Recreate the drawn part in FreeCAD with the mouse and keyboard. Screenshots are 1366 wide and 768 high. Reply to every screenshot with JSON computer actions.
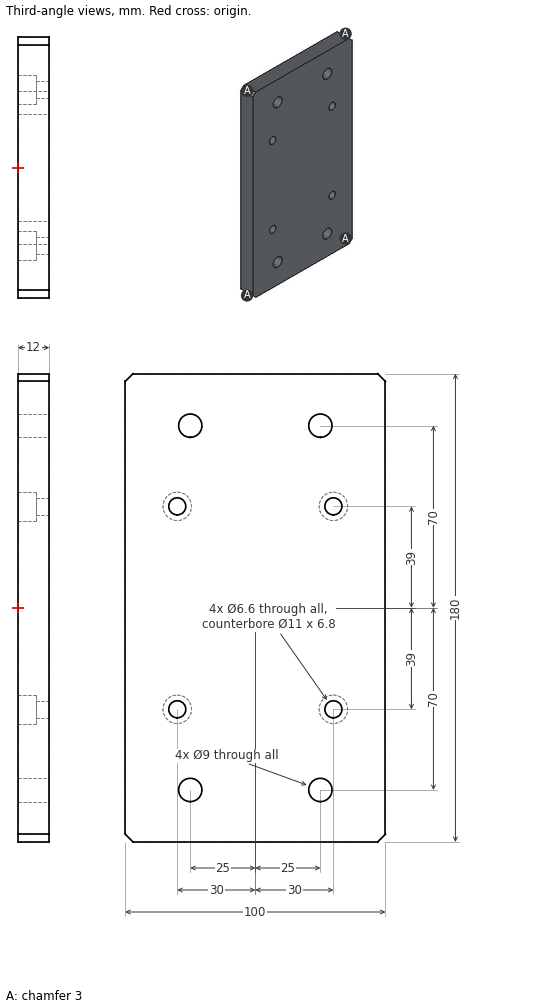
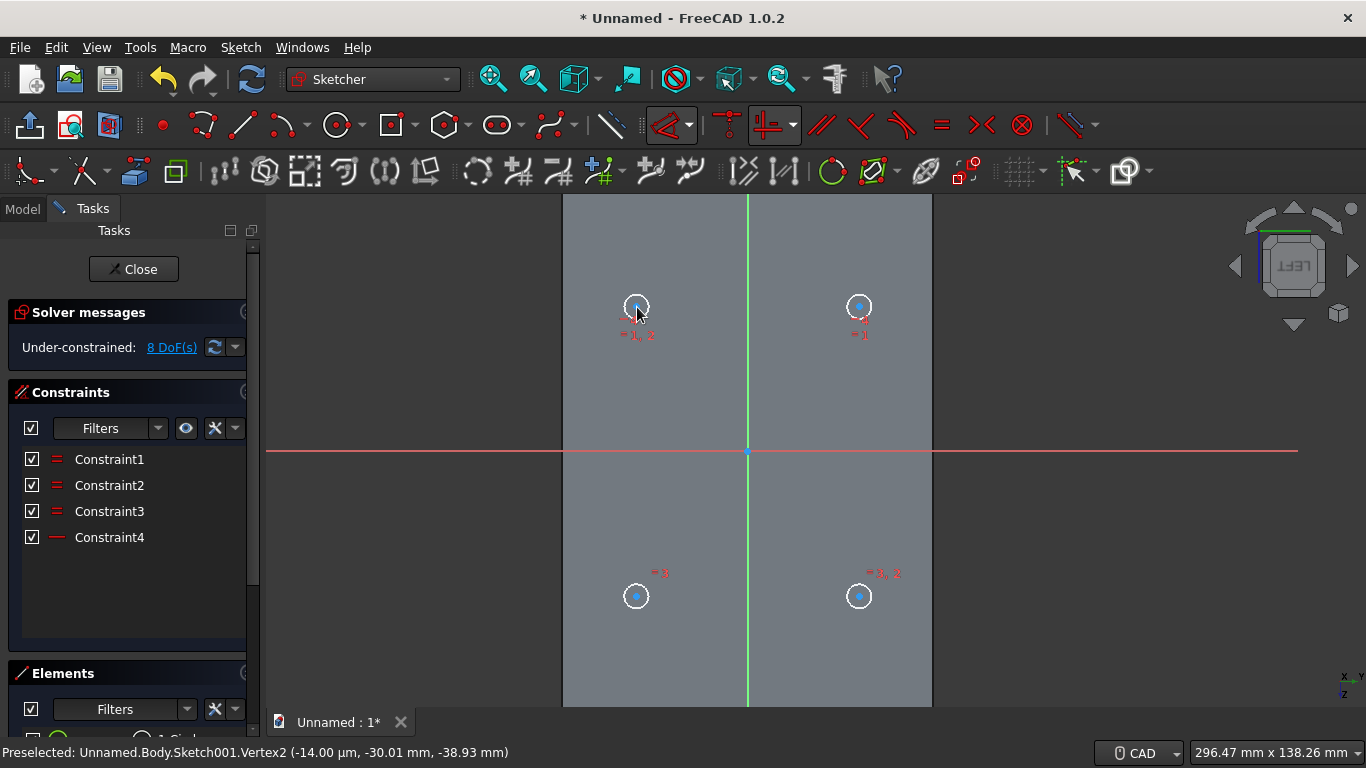
{"action": "left_click", "coordinate": [859, 307]}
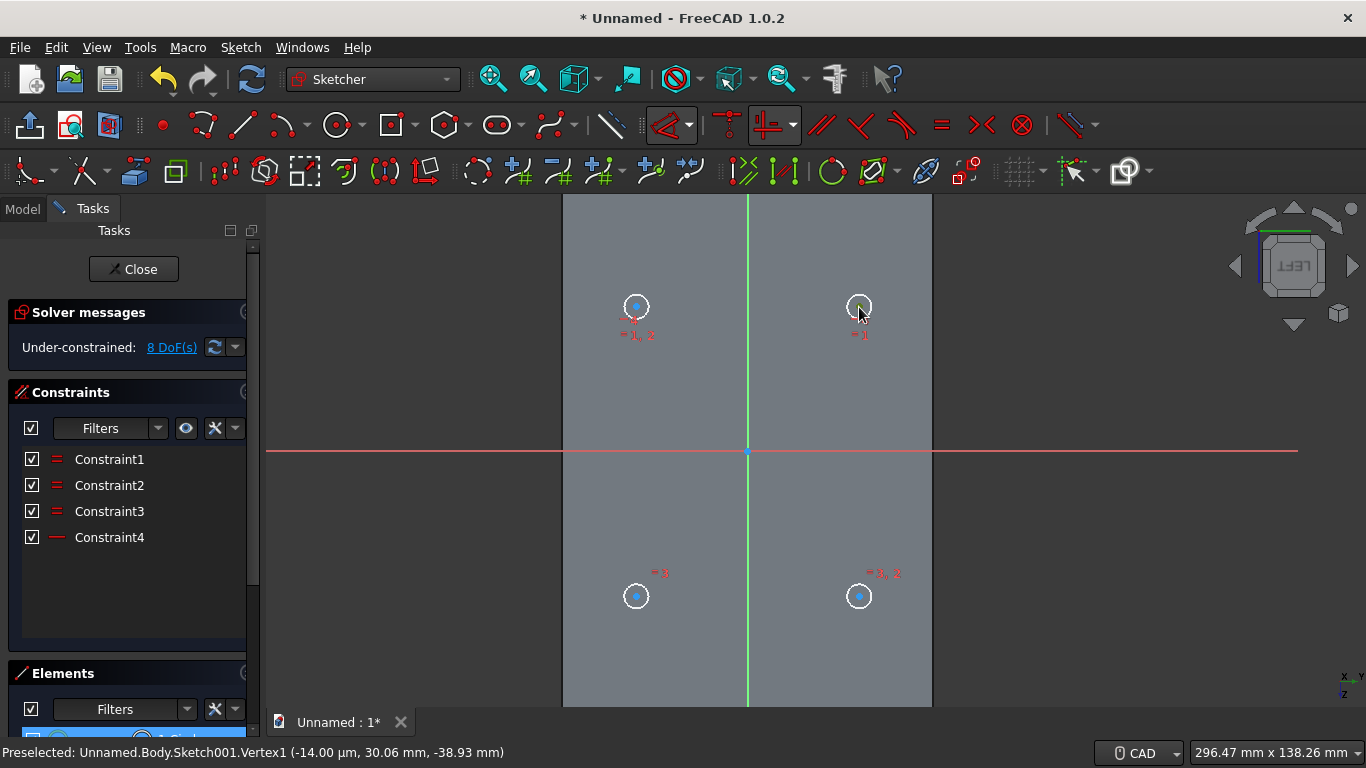
{"action": "left_click", "coordinate": [859, 596]}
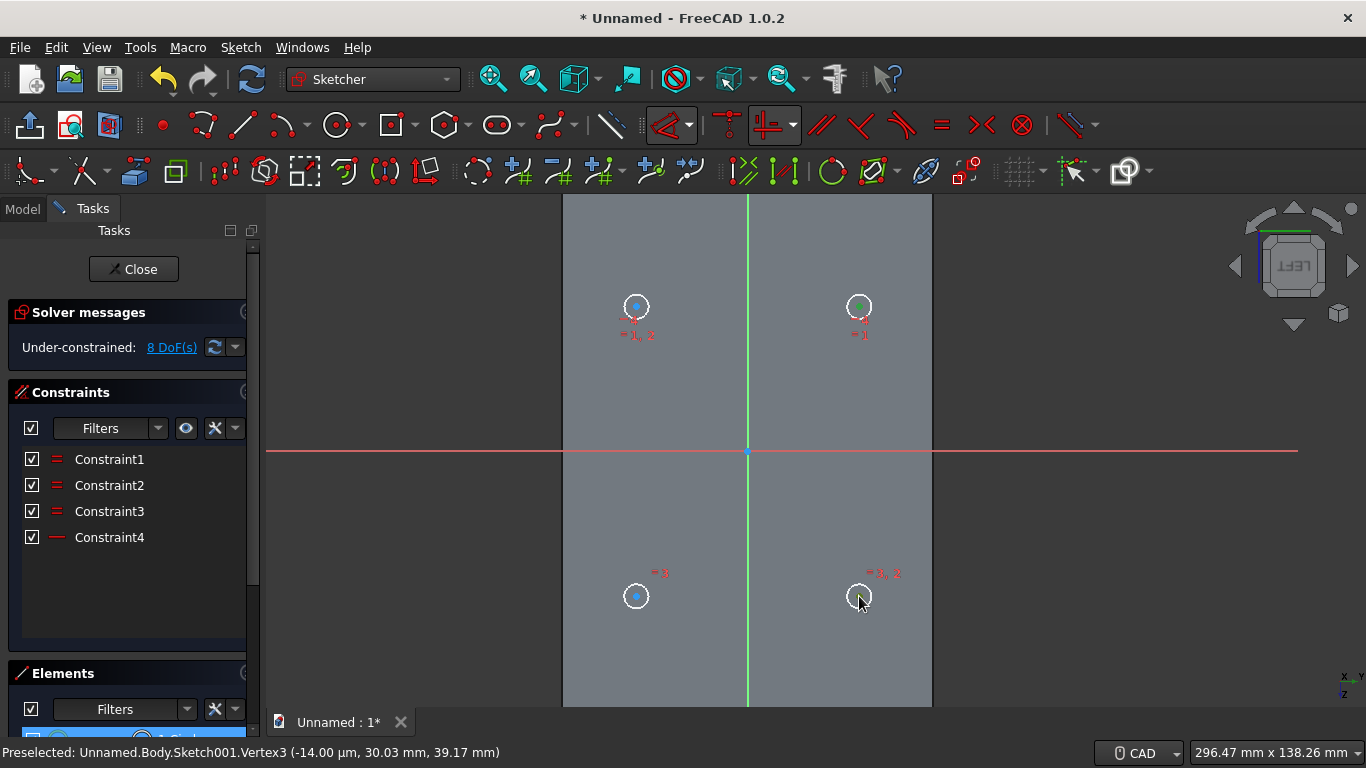
{"action": "left_click", "coordinate": [796, 126]}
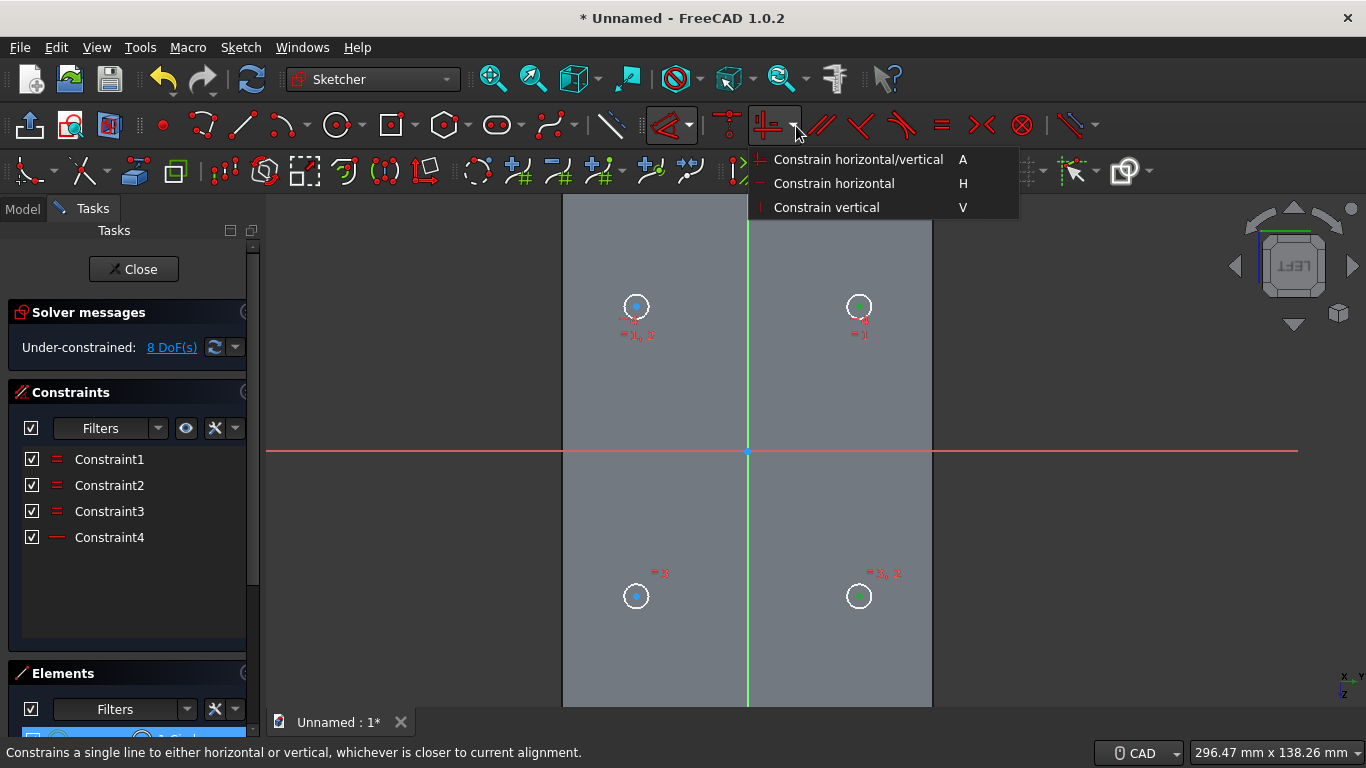
{"action": "left_click", "coordinate": [884, 207]}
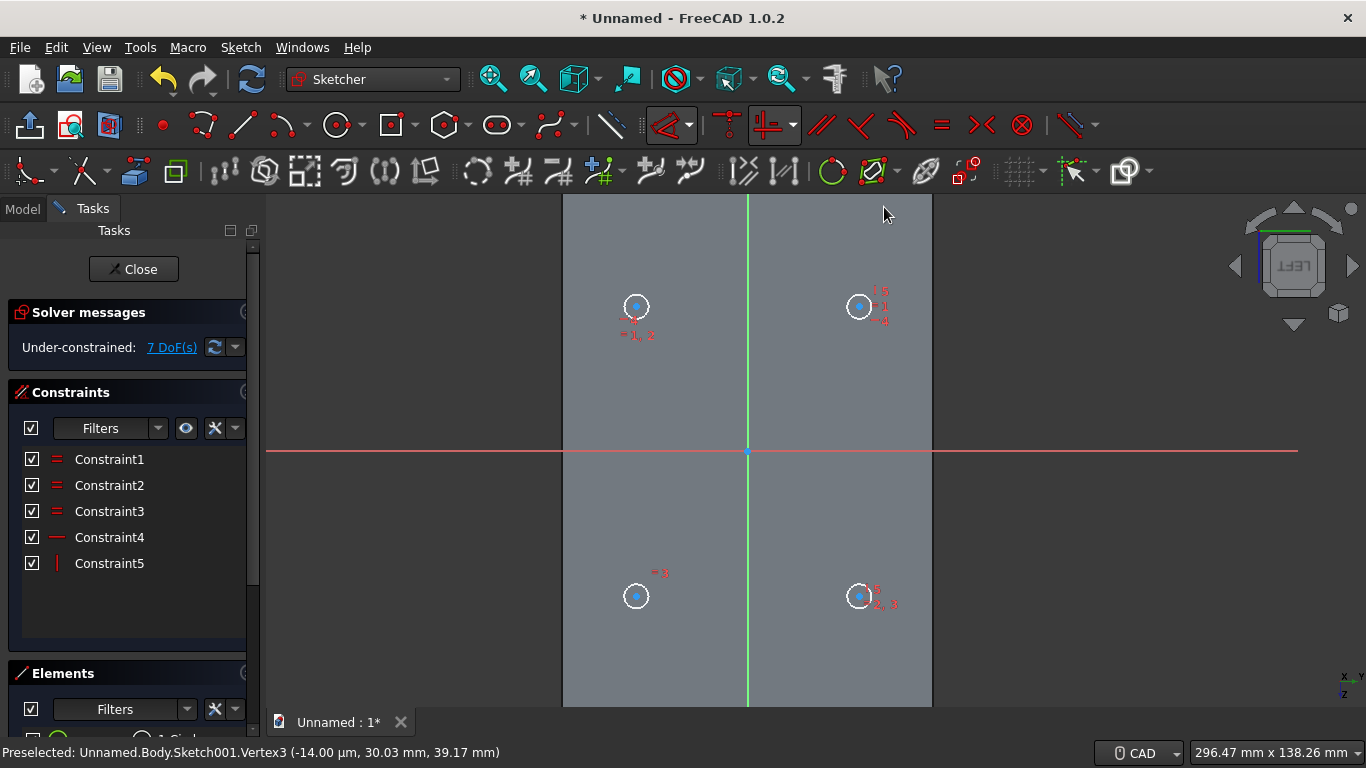
{"action": "left_click", "coordinate": [637, 307]}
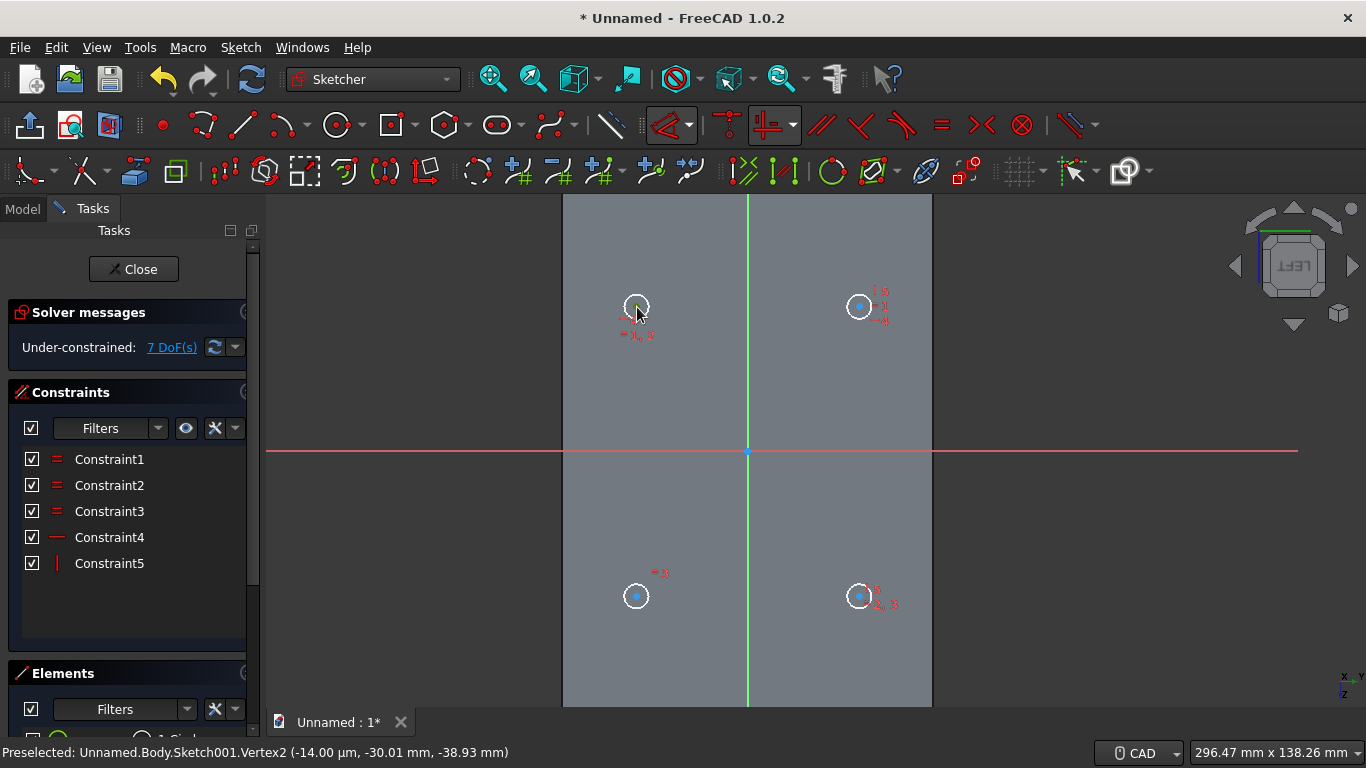
{"action": "left_click", "coordinate": [636, 596]}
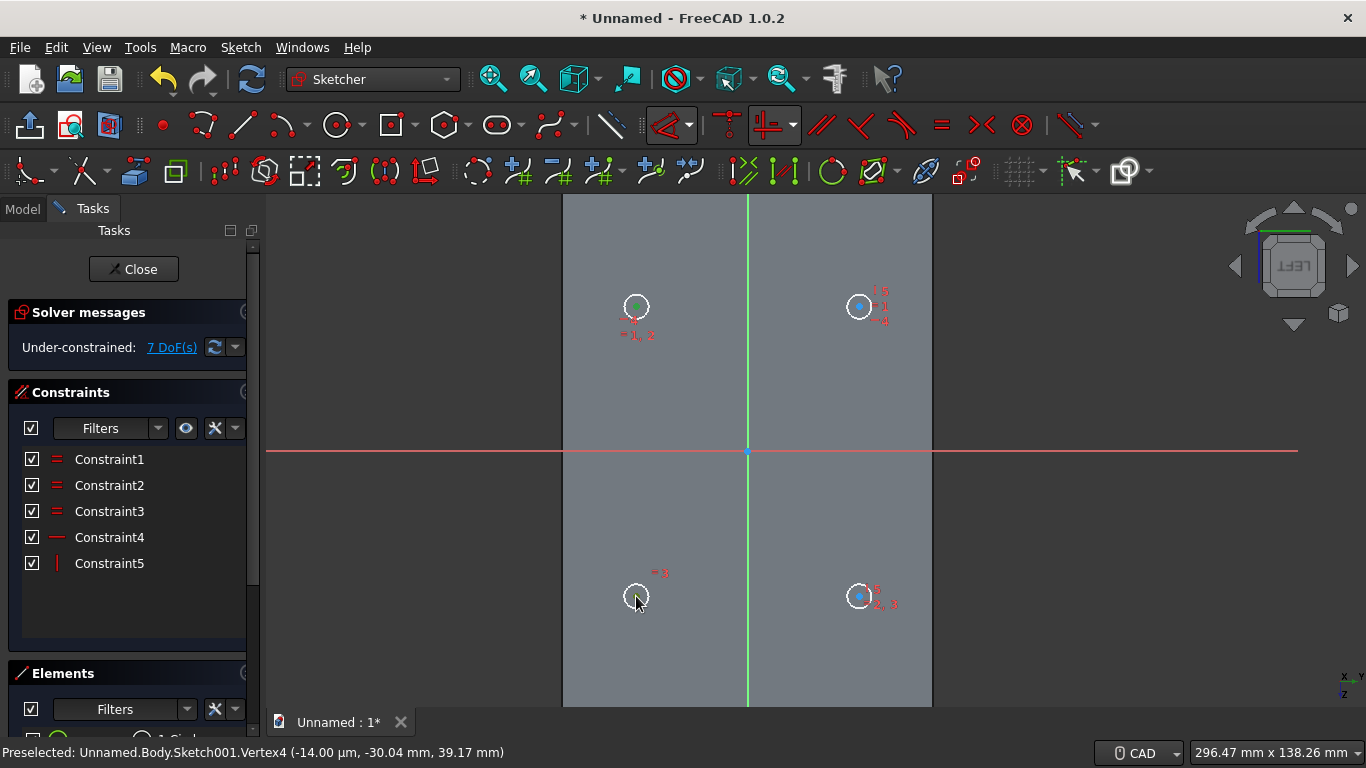
{"action": "key", "text": "v"}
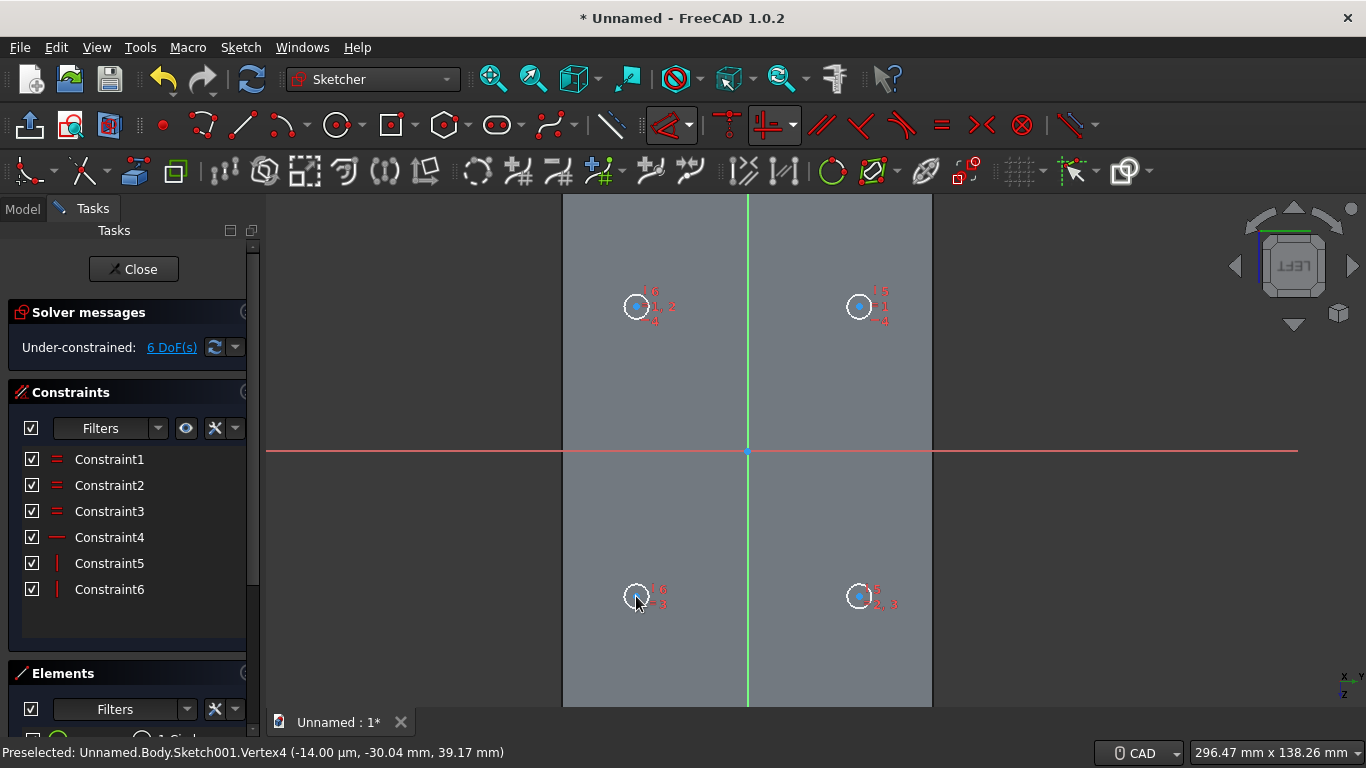
{"action": "left_click", "coordinate": [859, 596]}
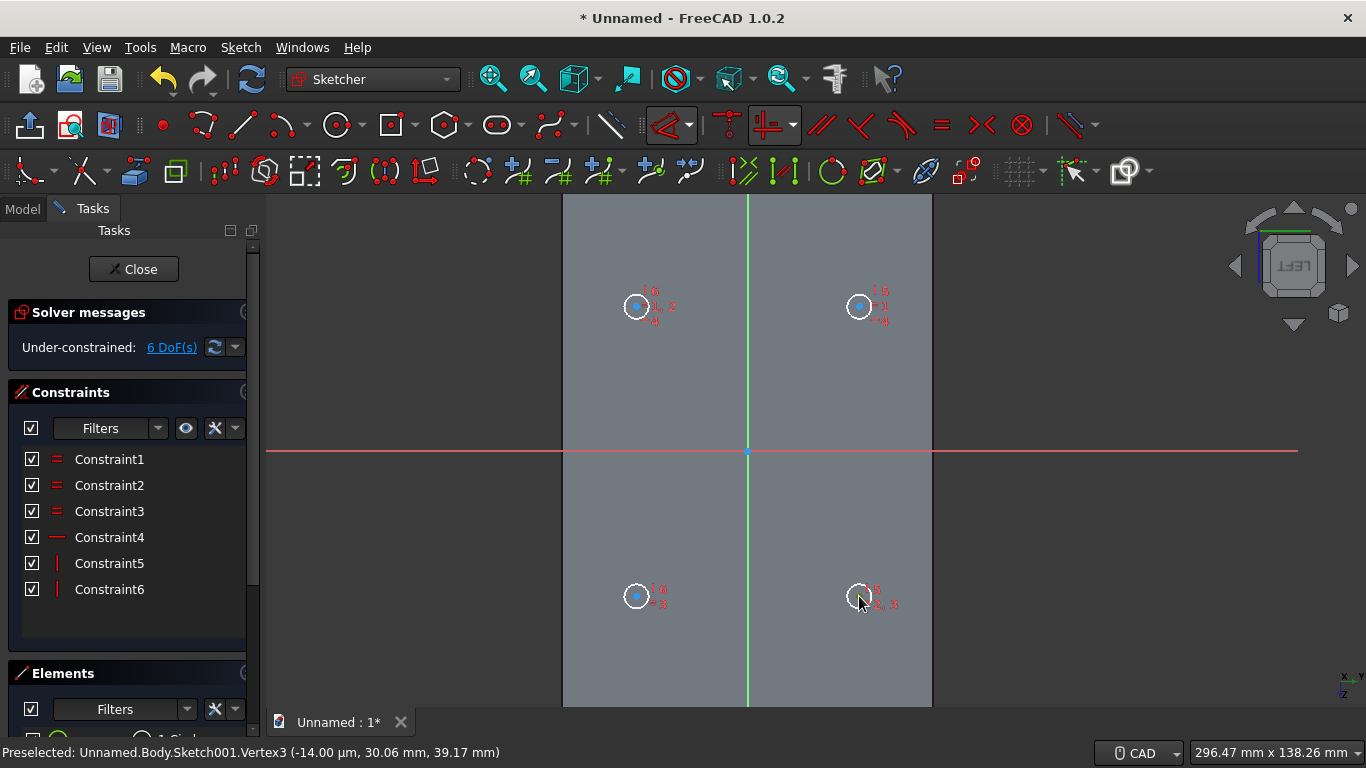
{"action": "left_click", "coordinate": [637, 596]}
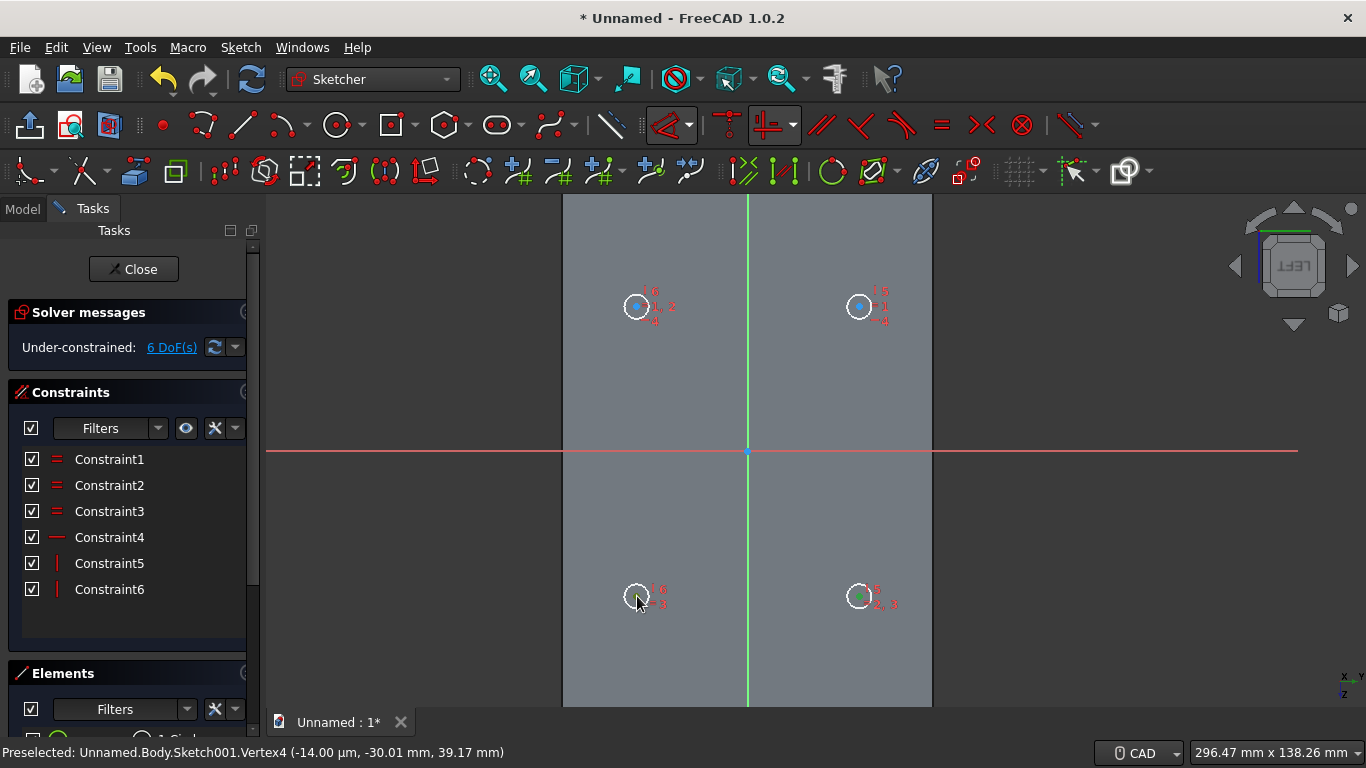
{"action": "key", "text": "h"}